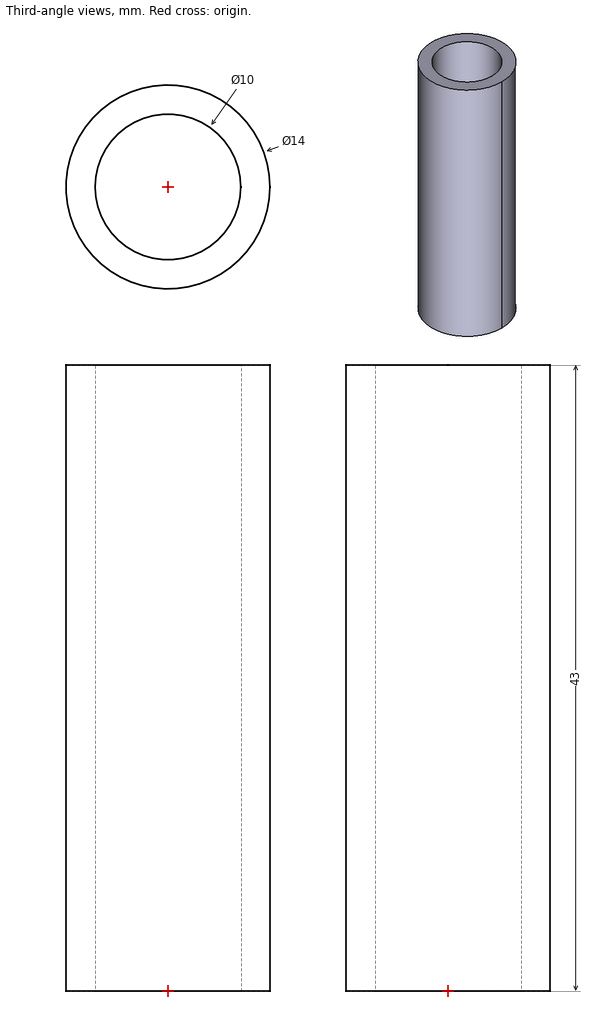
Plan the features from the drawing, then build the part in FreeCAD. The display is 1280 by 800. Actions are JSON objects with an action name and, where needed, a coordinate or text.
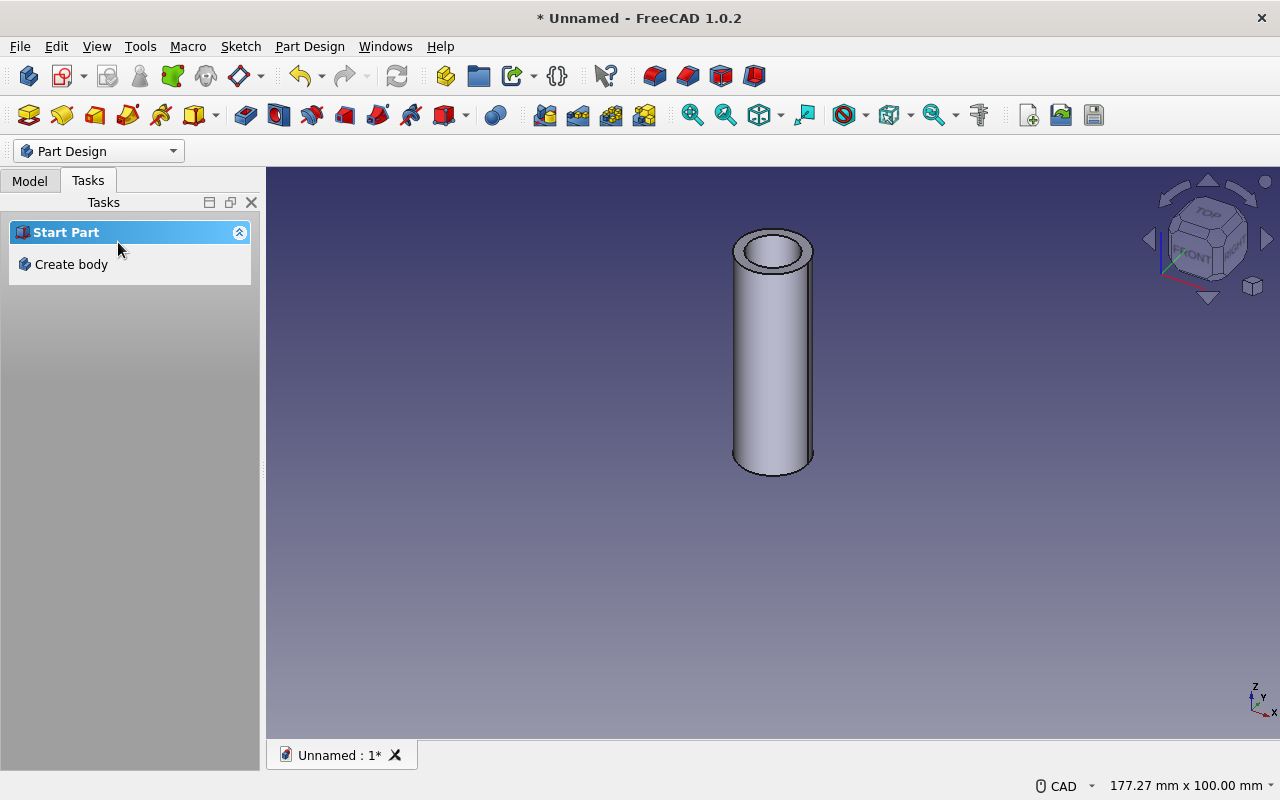
{"action": "key", "text": "0"}